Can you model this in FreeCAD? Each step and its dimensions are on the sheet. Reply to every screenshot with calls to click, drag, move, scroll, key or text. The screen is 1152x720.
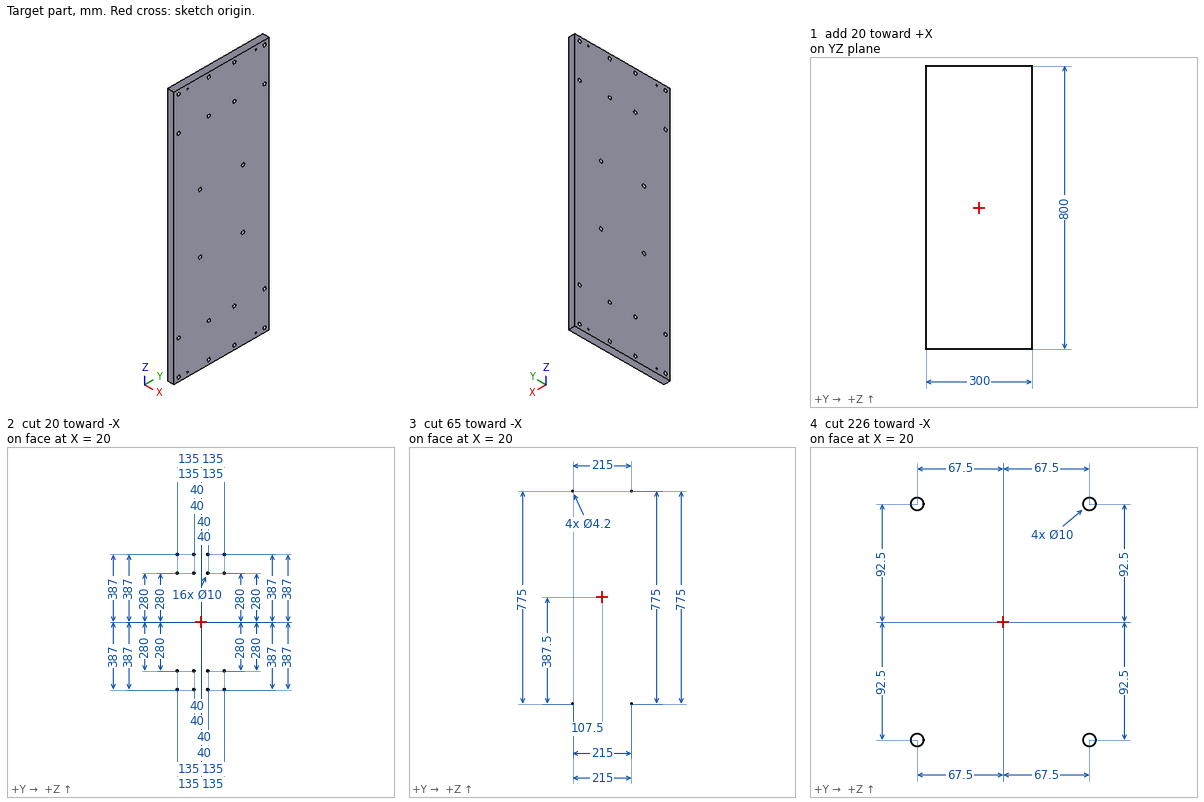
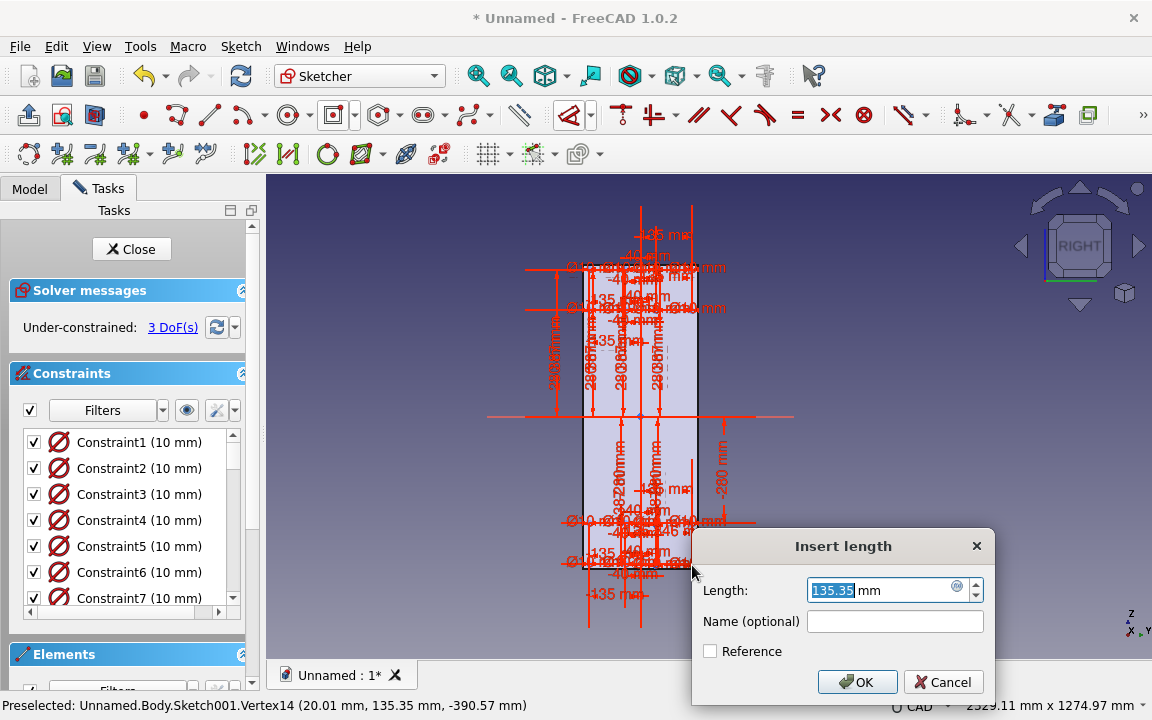
text(135)
key(Return)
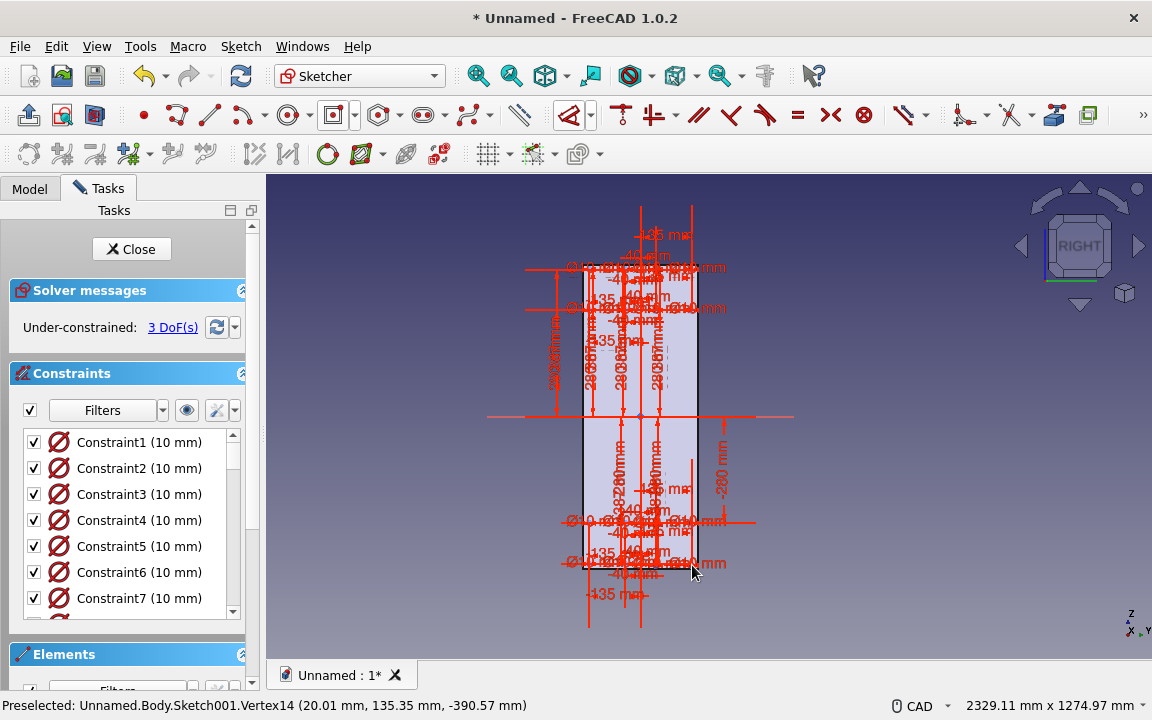
click(692, 565)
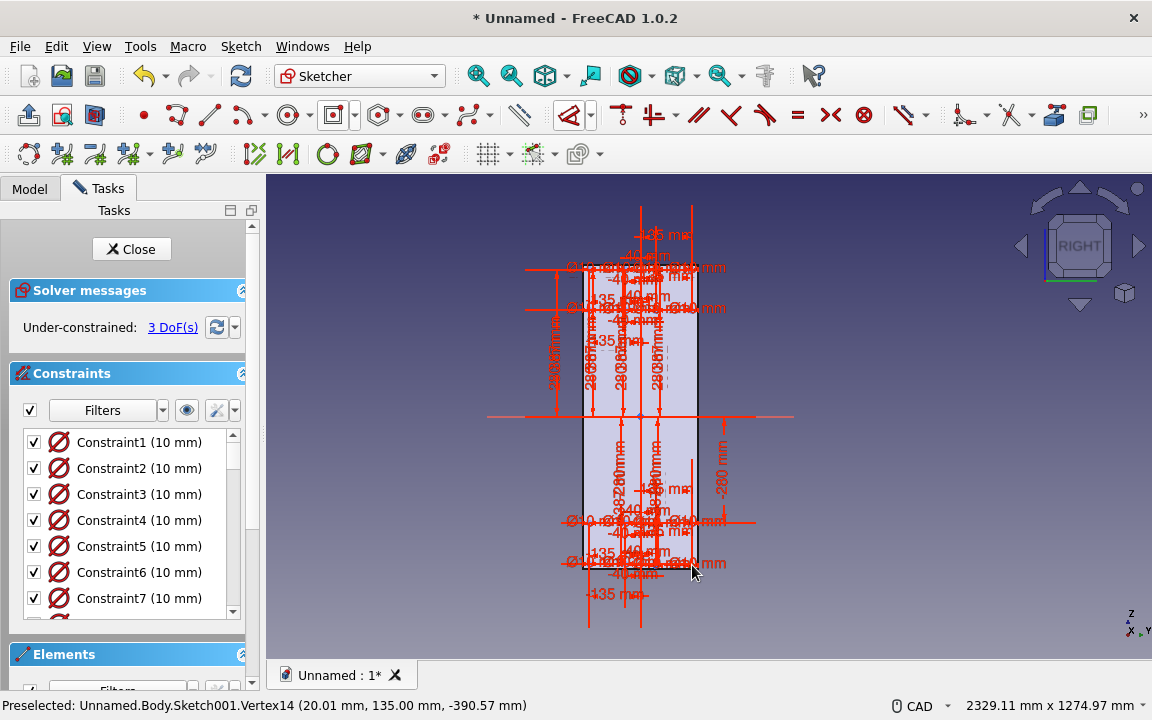
key(i)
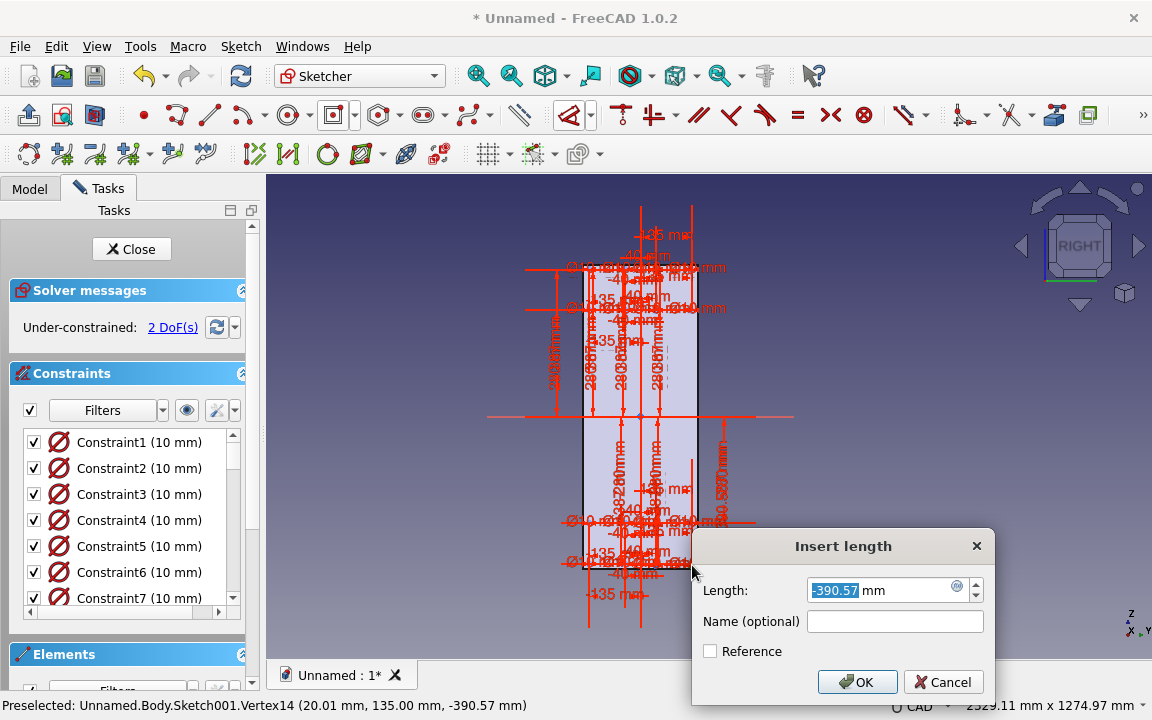
text(-387)
key(Return)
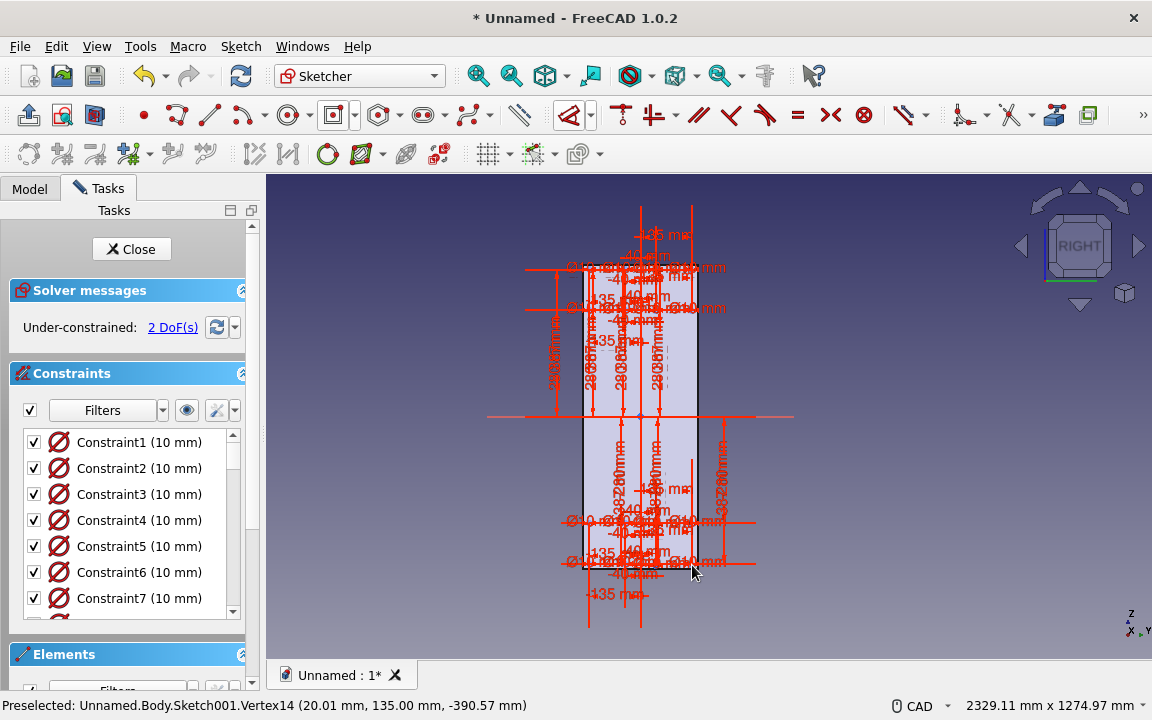
click(656, 565)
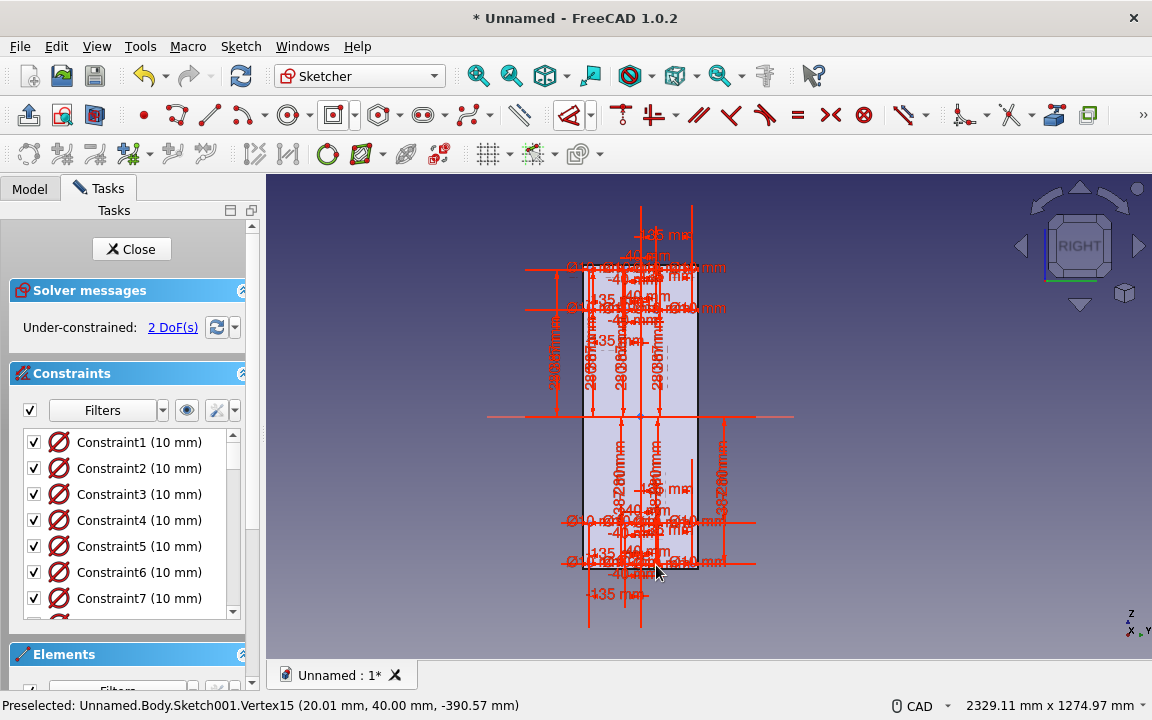
key(i)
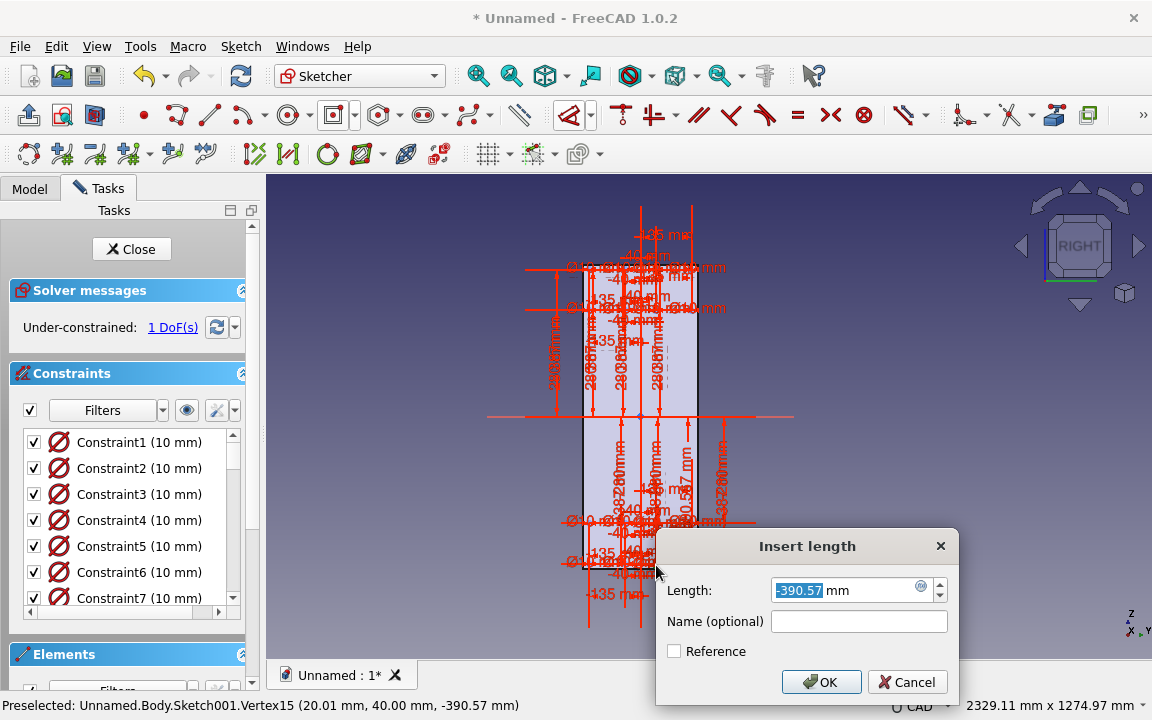
text(-387)
key(Return)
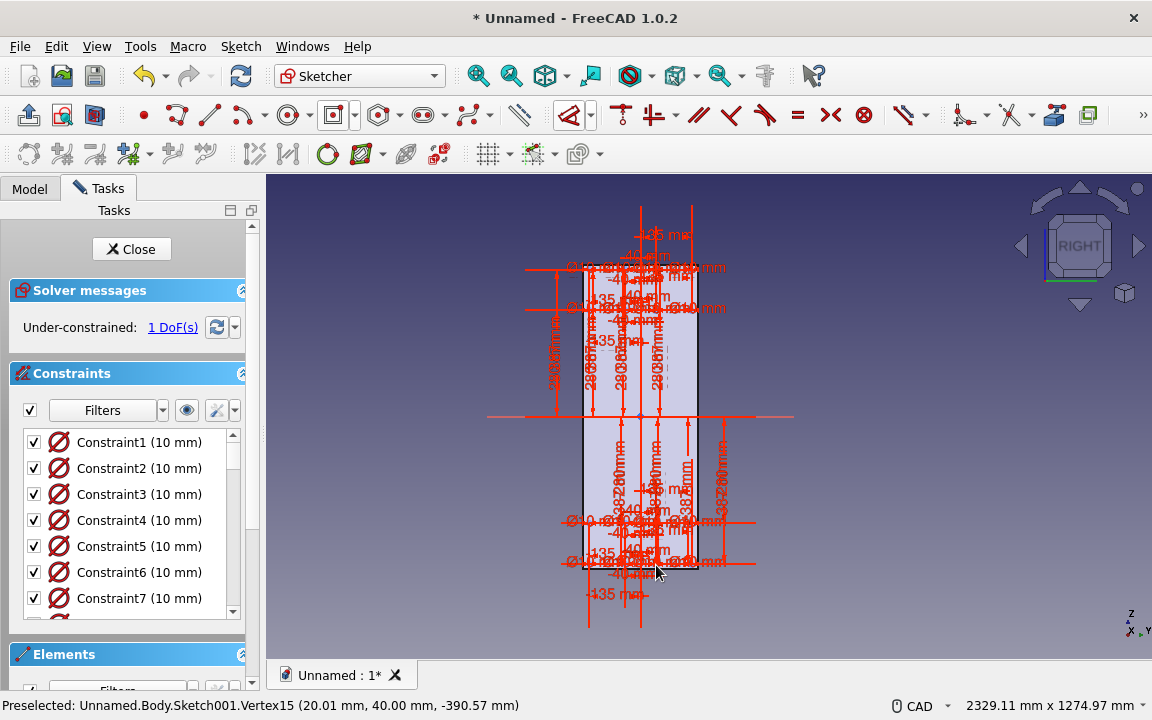
click(656, 524)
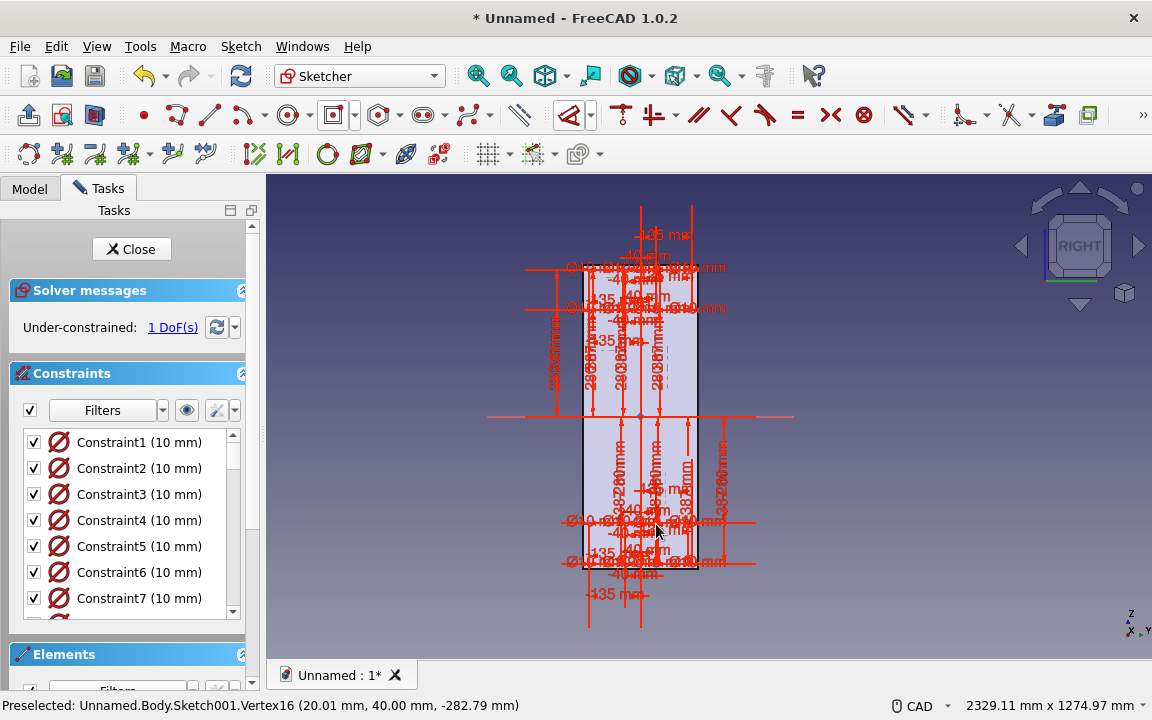
key(i)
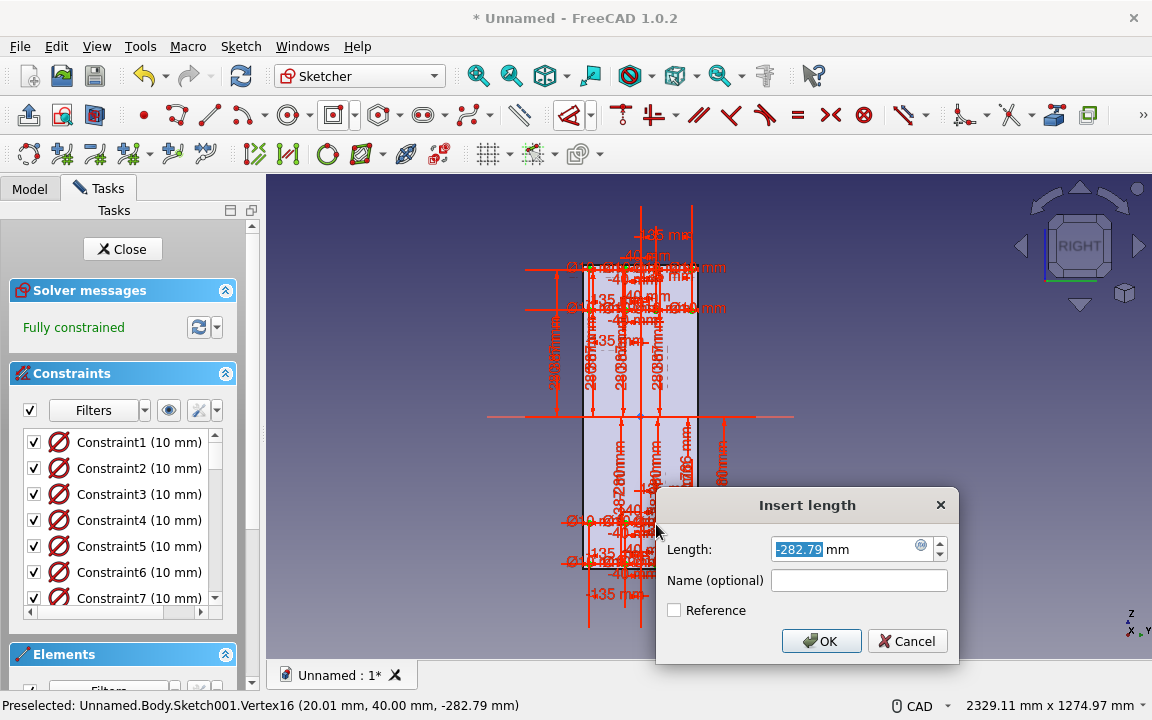
text(-280)
key(Return)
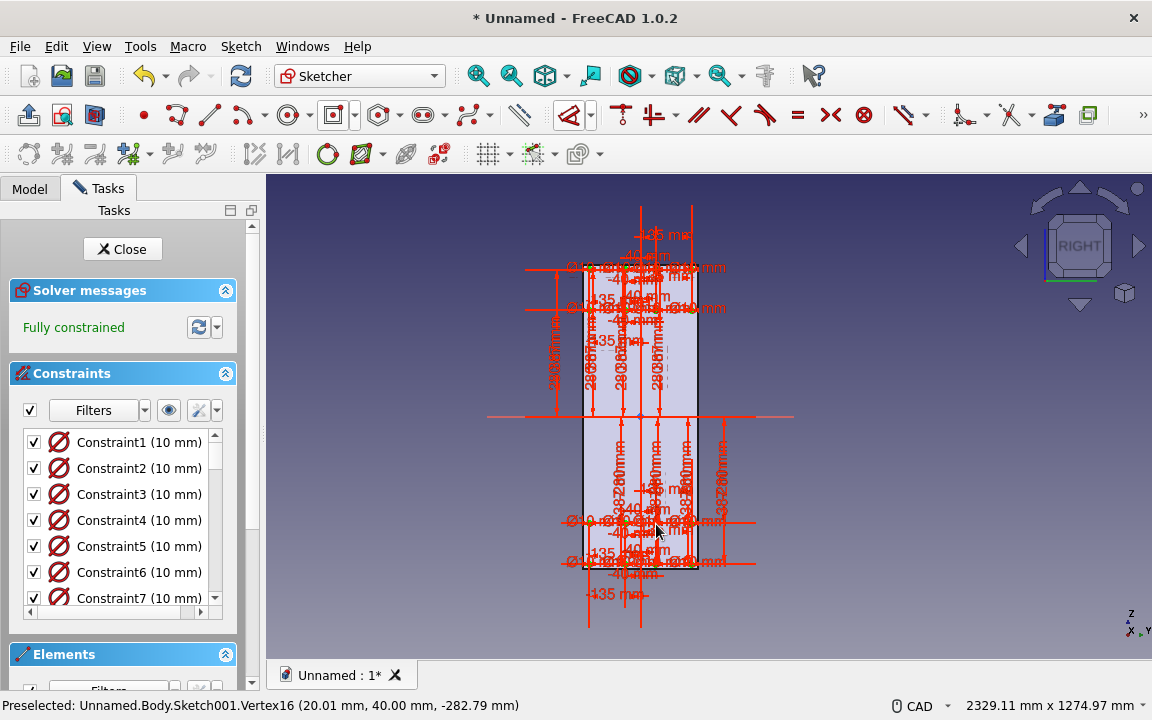
click(123, 249)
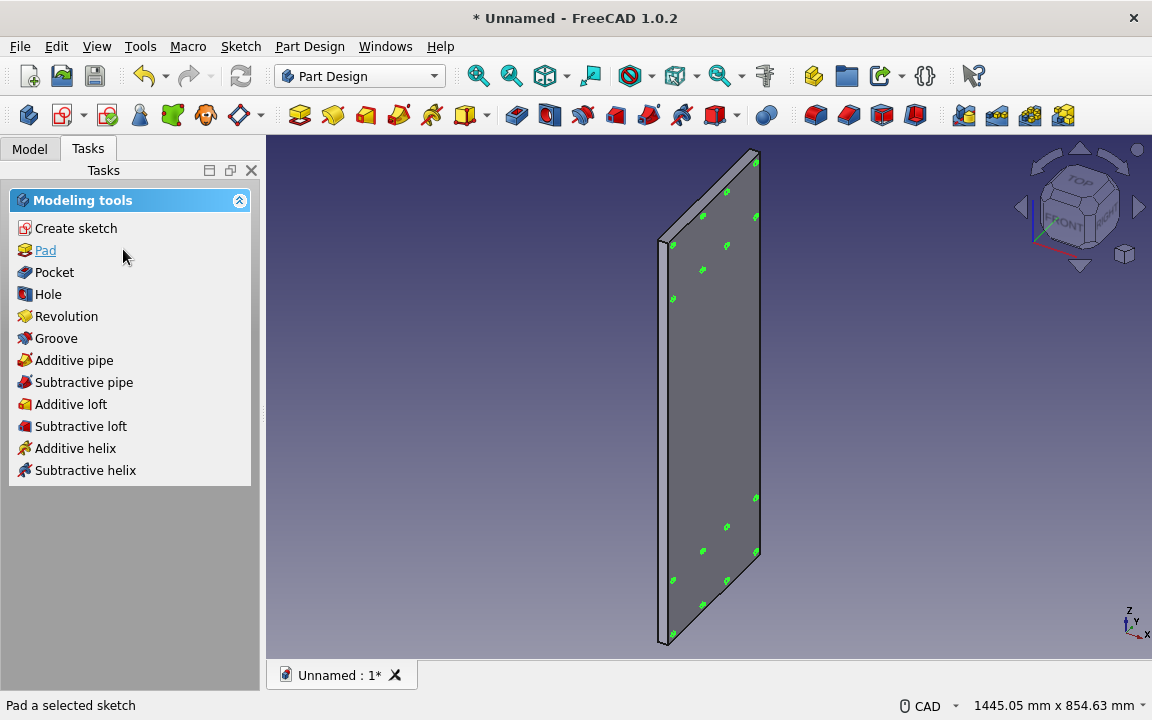
click(517, 116)